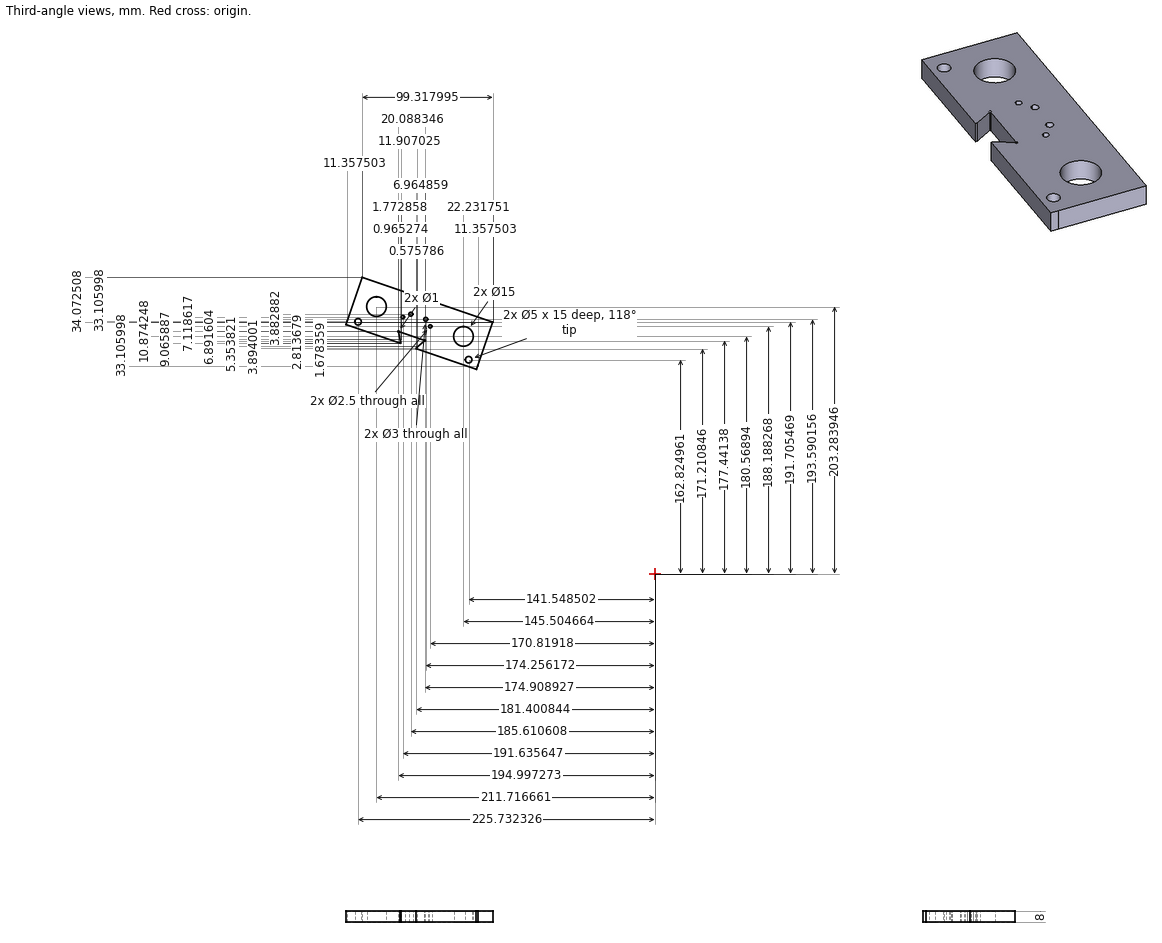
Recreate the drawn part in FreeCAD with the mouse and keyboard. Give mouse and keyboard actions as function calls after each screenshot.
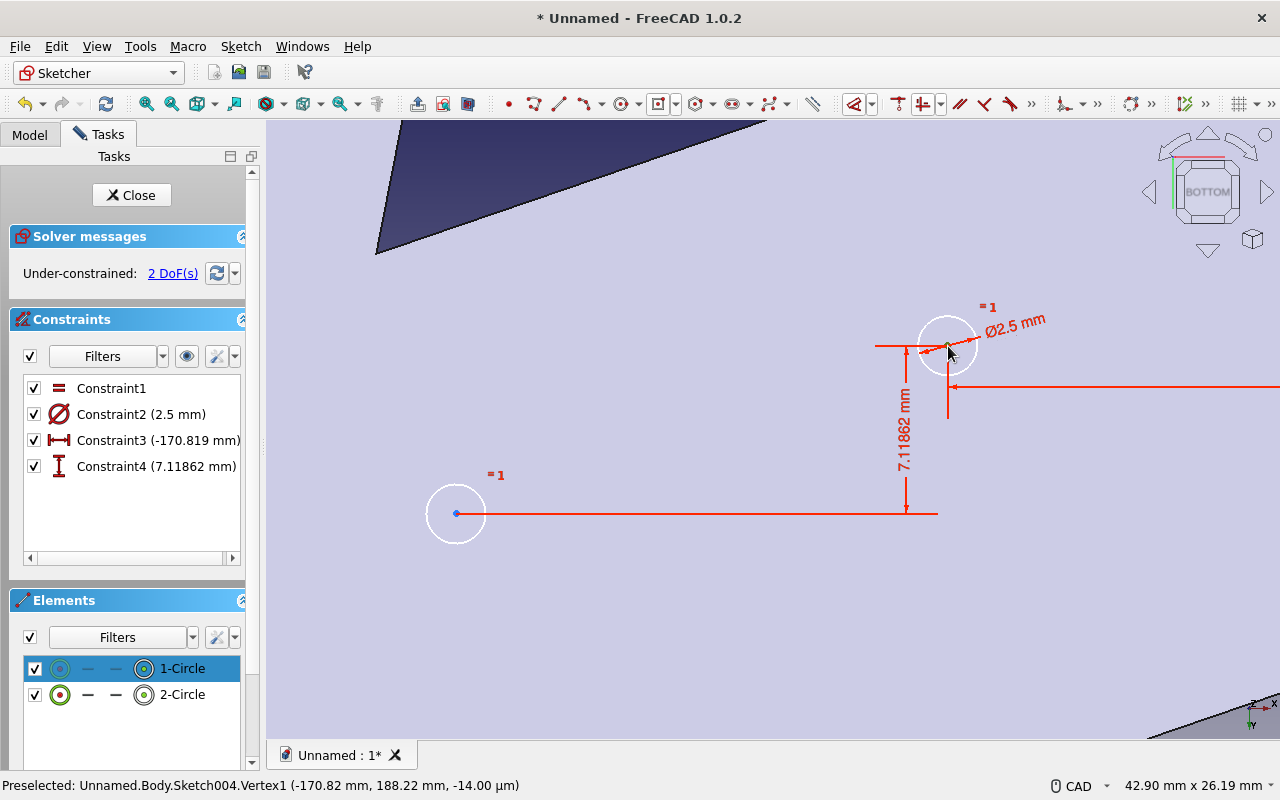
click(872, 104)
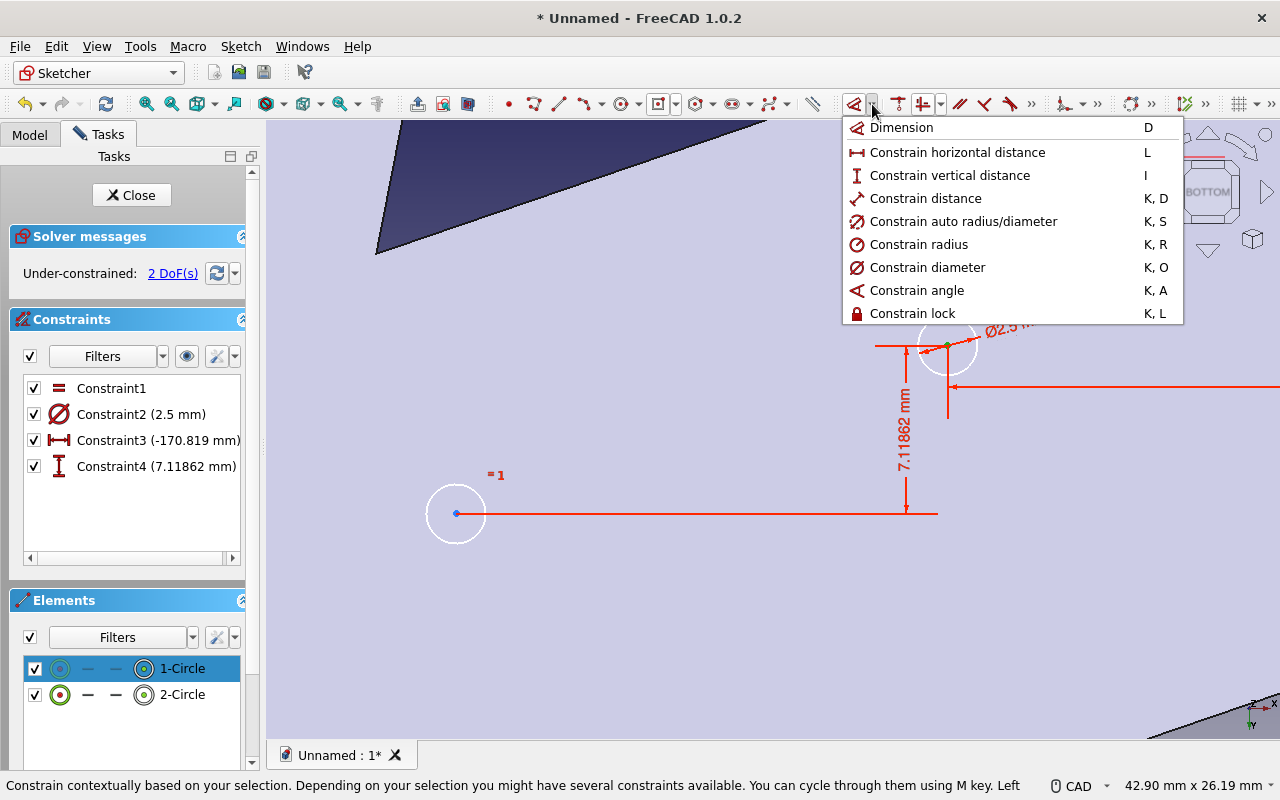
click(1013, 176)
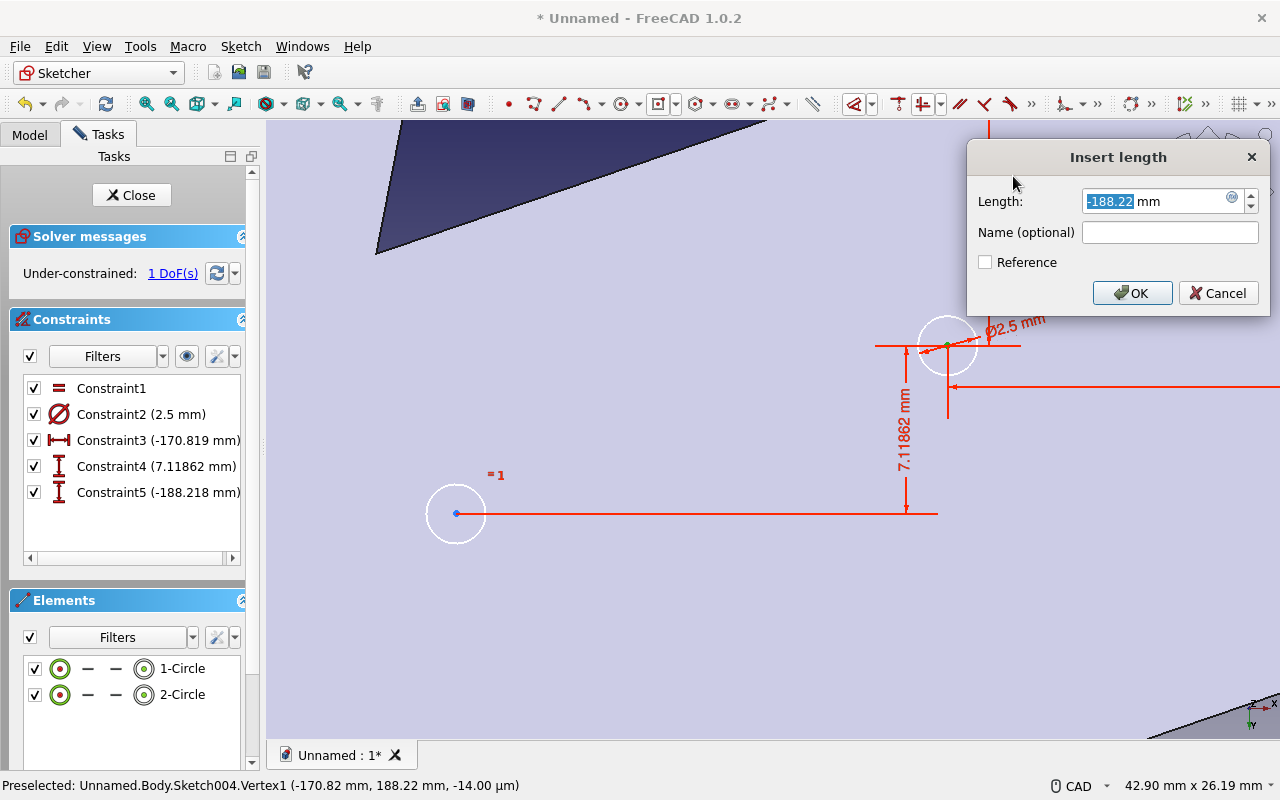
text(-188.188268)
key(Return)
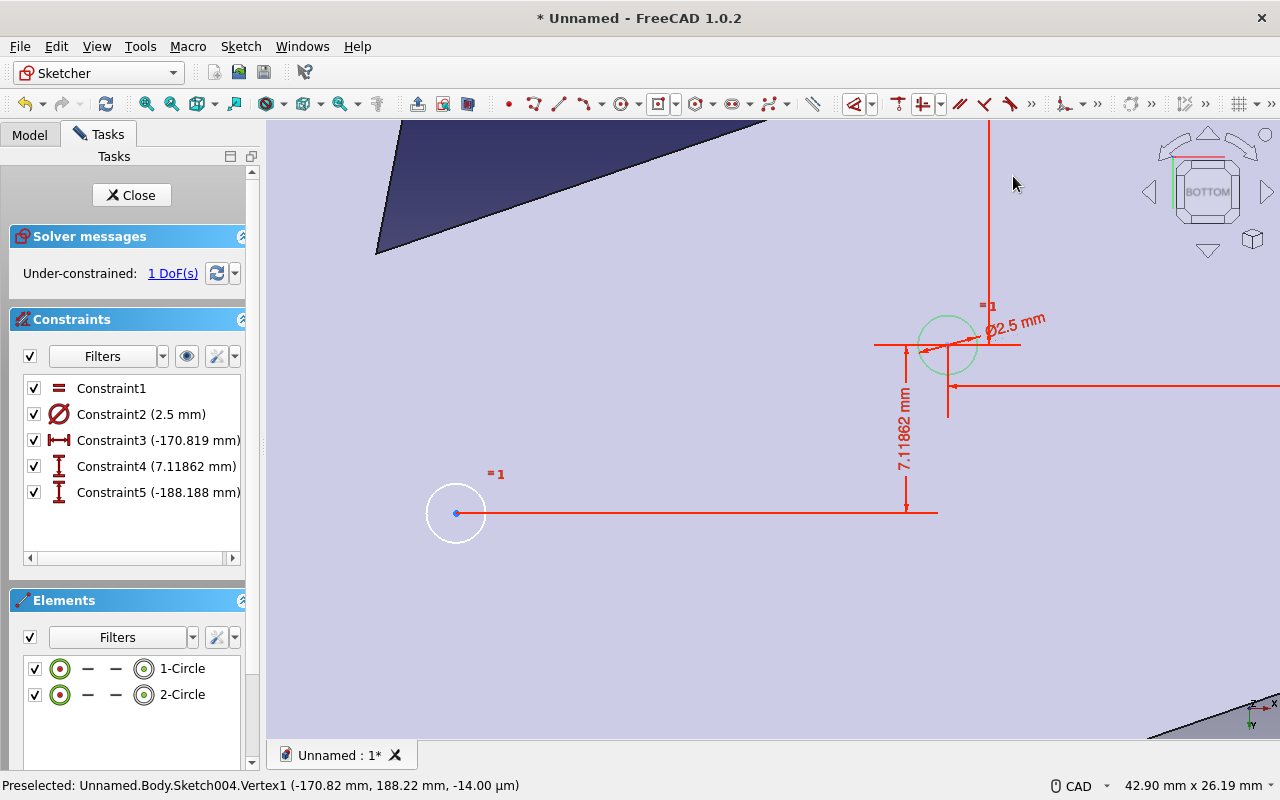
click(456, 513)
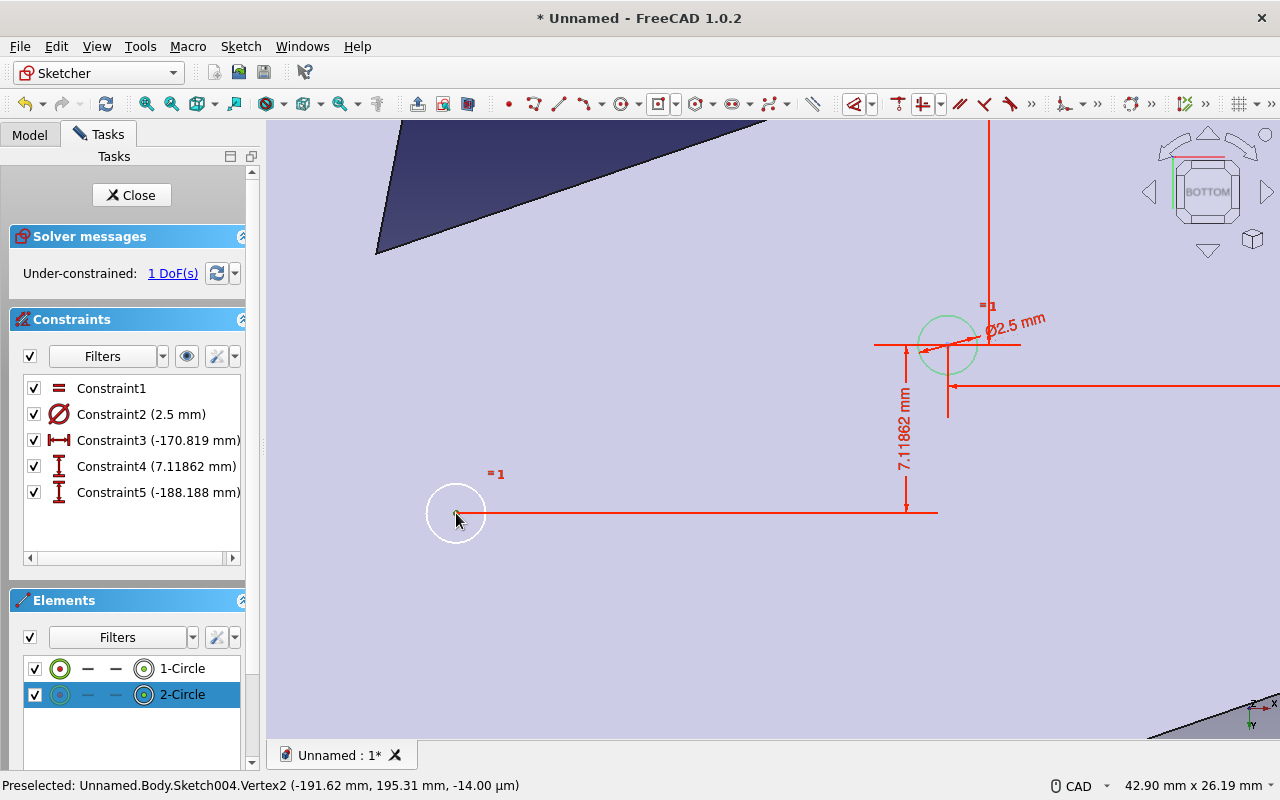
click(872, 104)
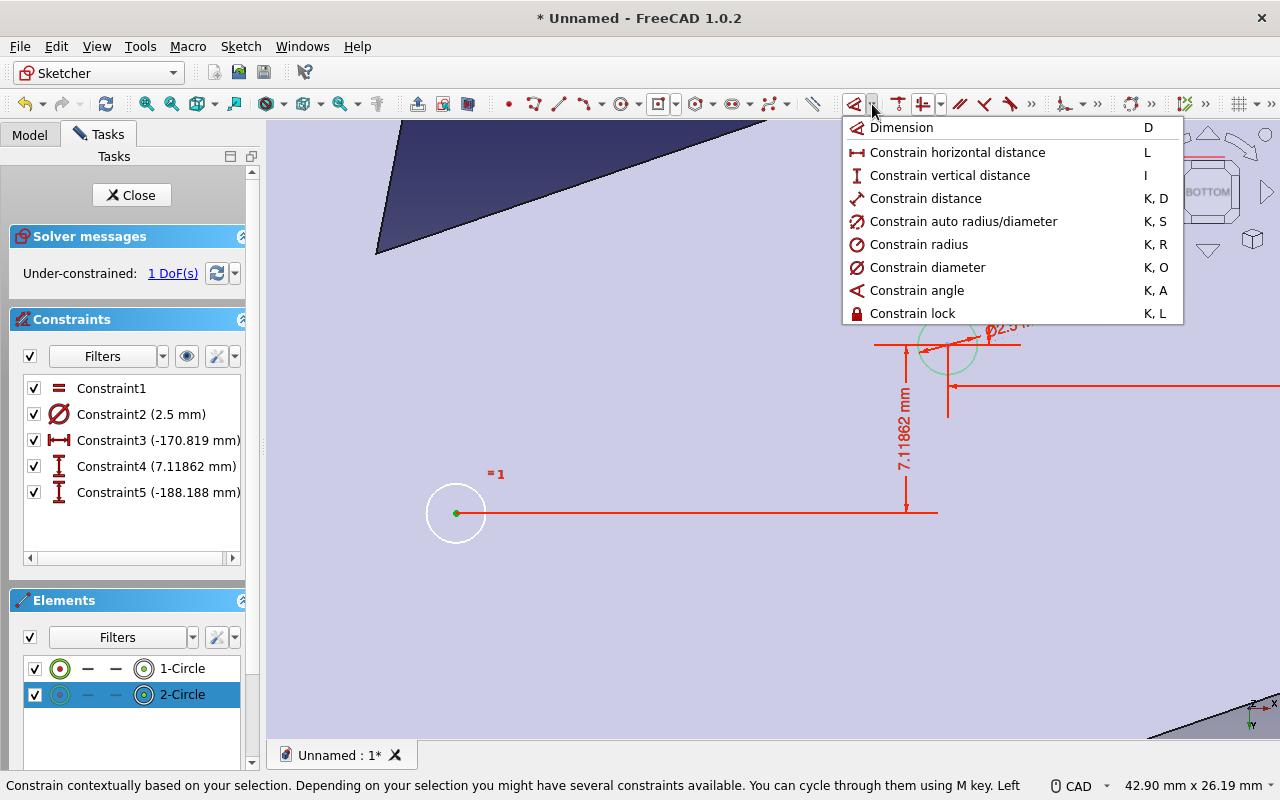
click(1013, 152)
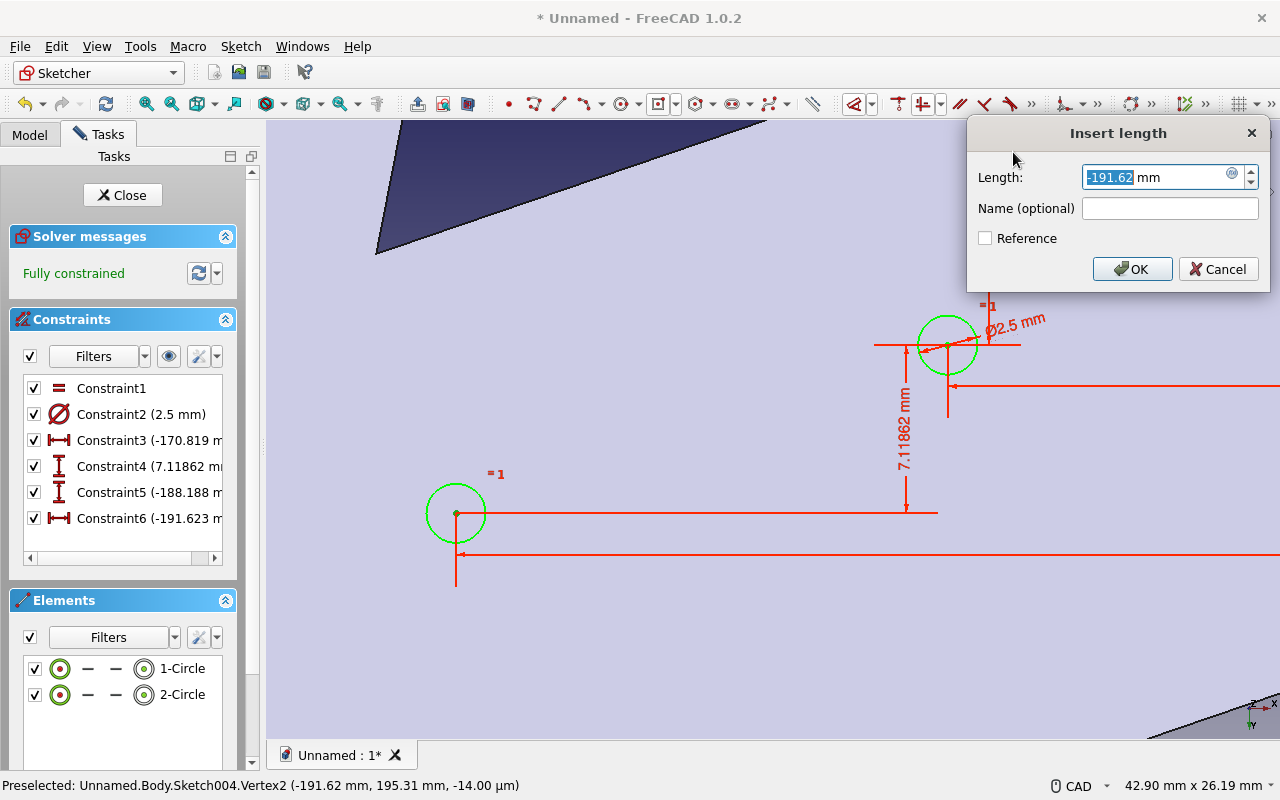
text(-191.635647)
key(Return)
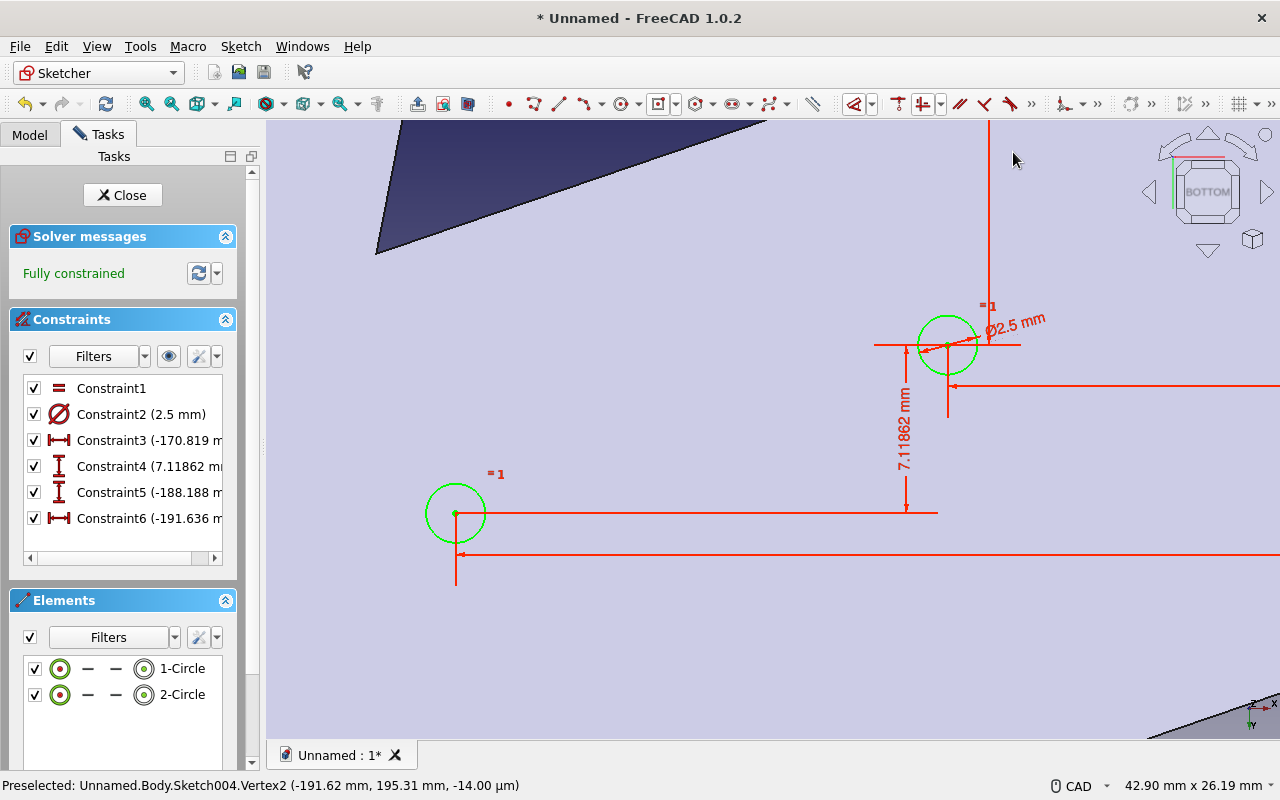
click(123, 195)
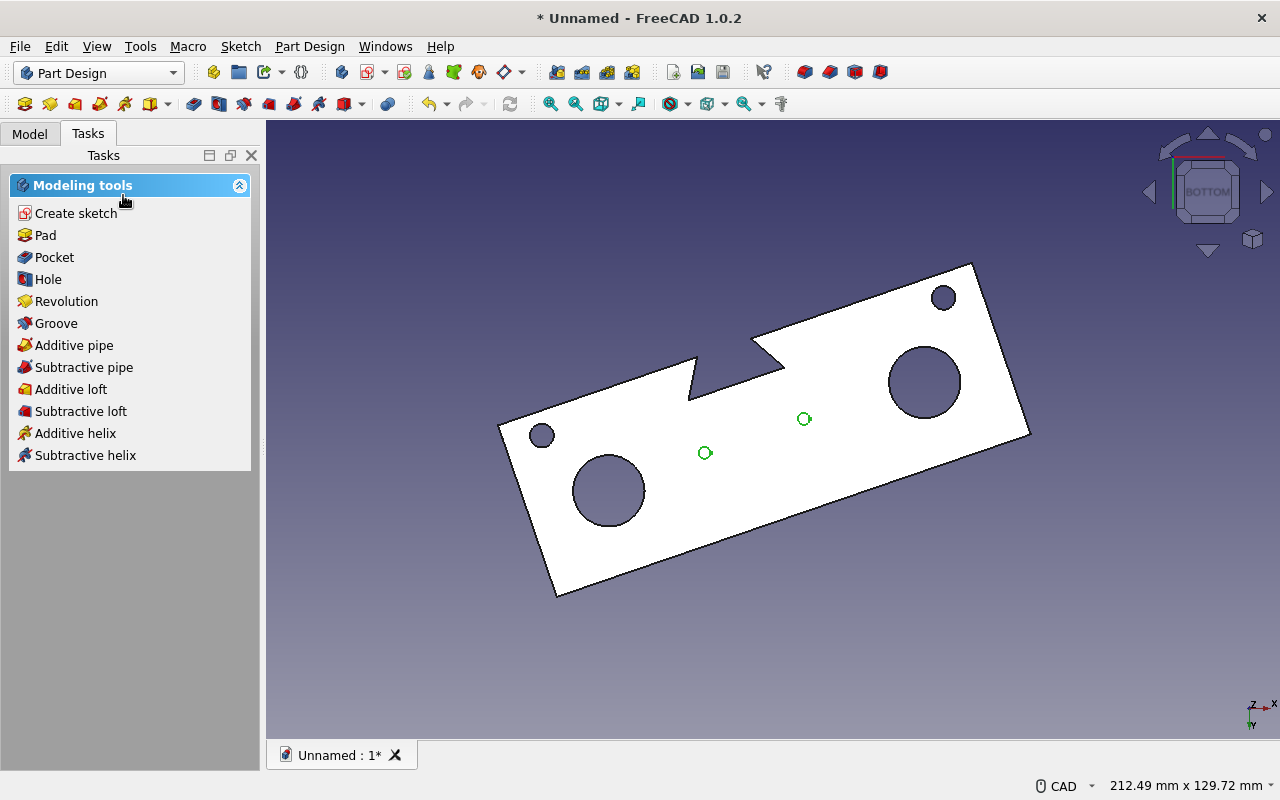
click(219, 104)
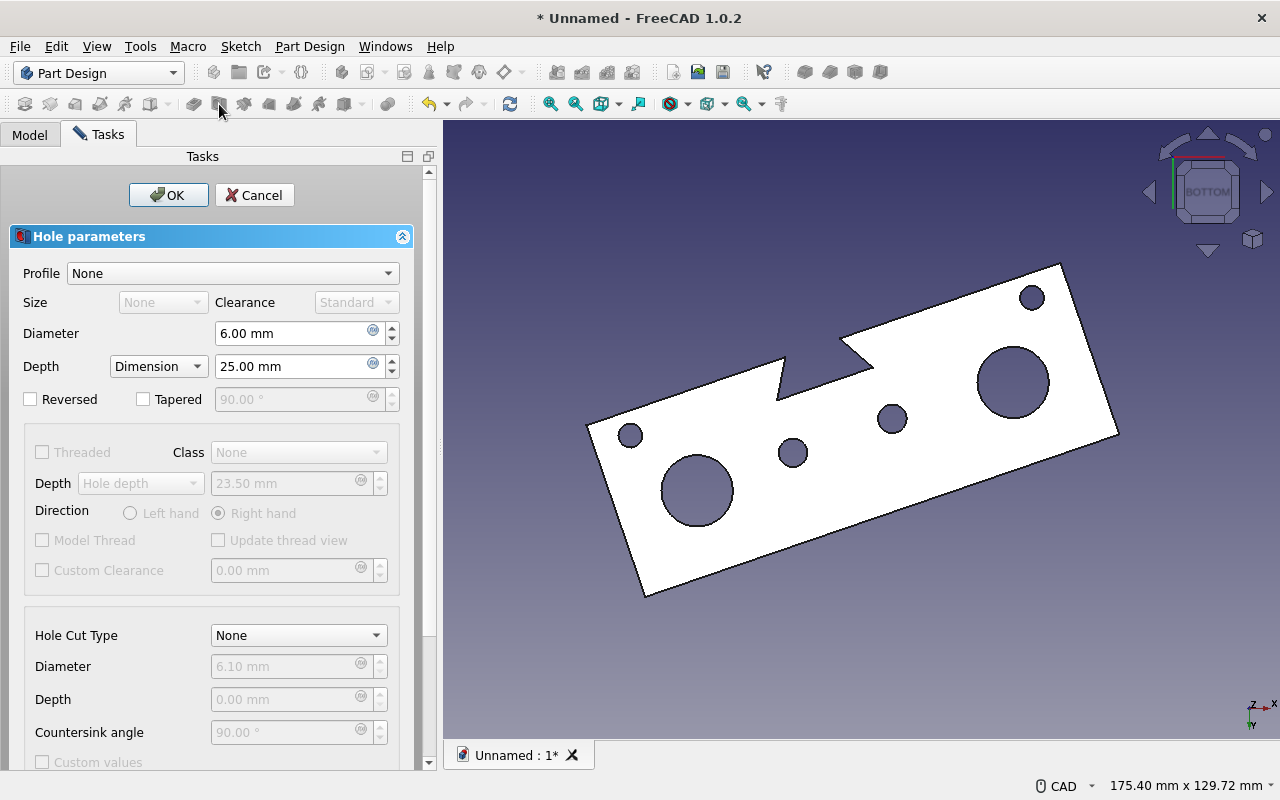
triple_click(300, 334)